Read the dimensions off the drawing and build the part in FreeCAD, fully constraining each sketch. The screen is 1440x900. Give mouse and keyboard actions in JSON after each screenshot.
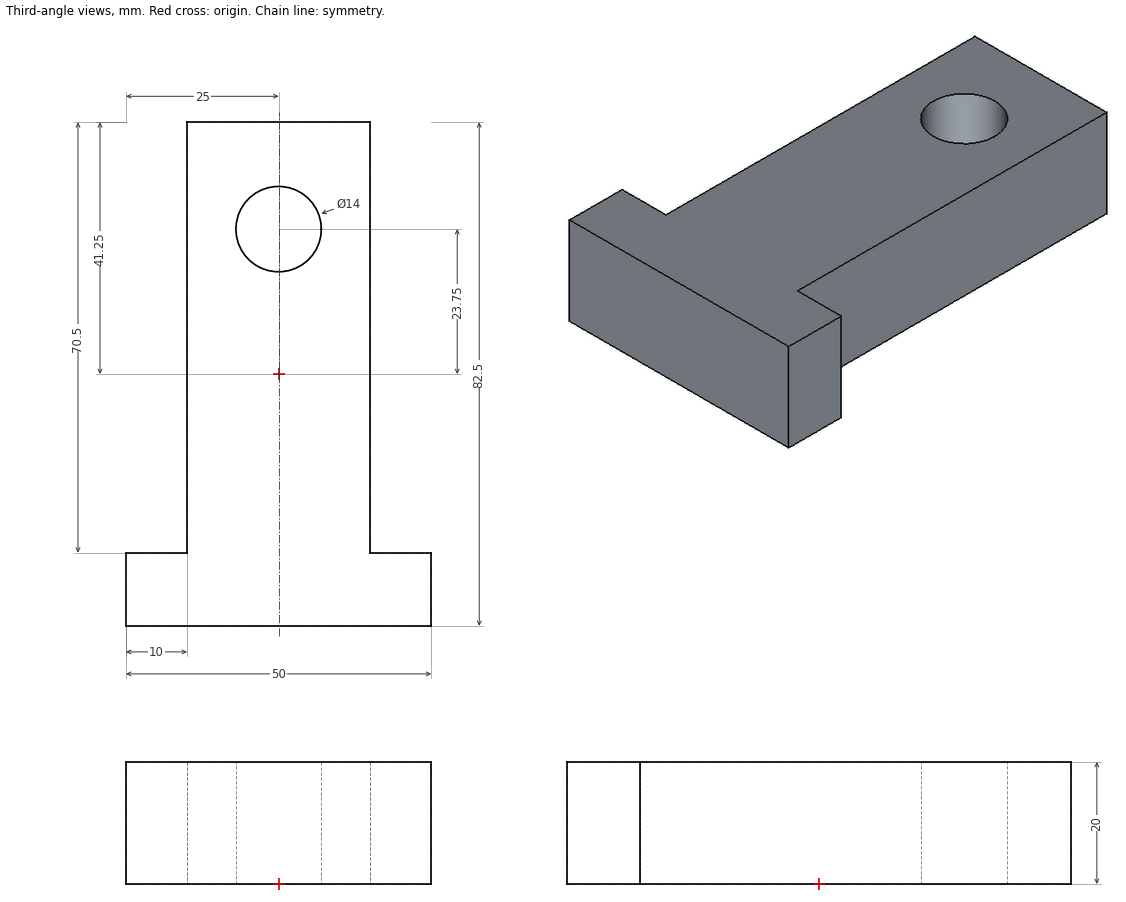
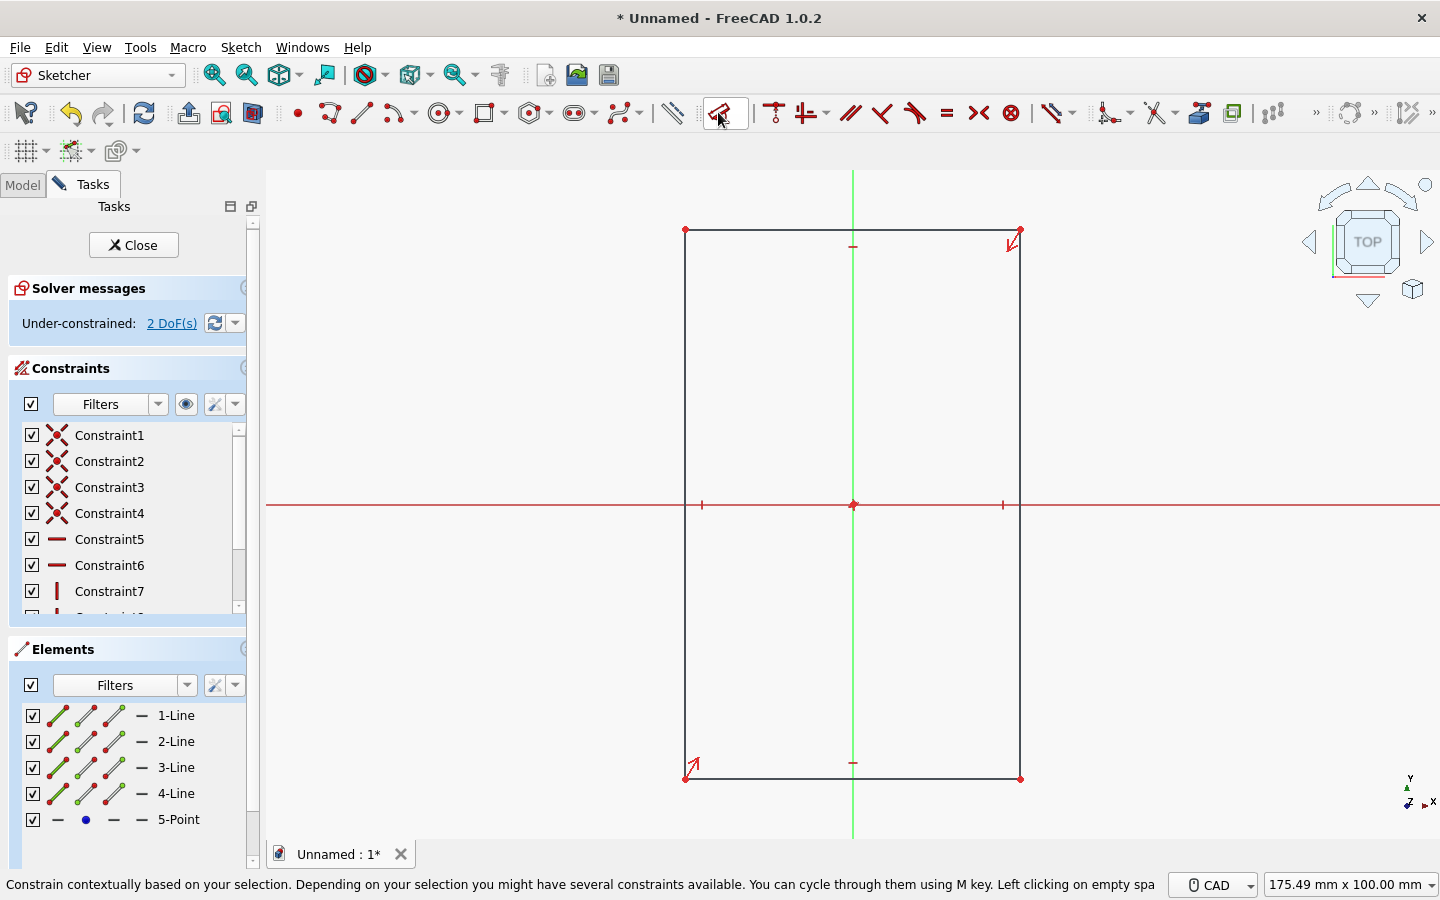
{"action": "left_click", "coordinate": [786, 779]}
{"action": "left_click", "coordinate": [776, 745]}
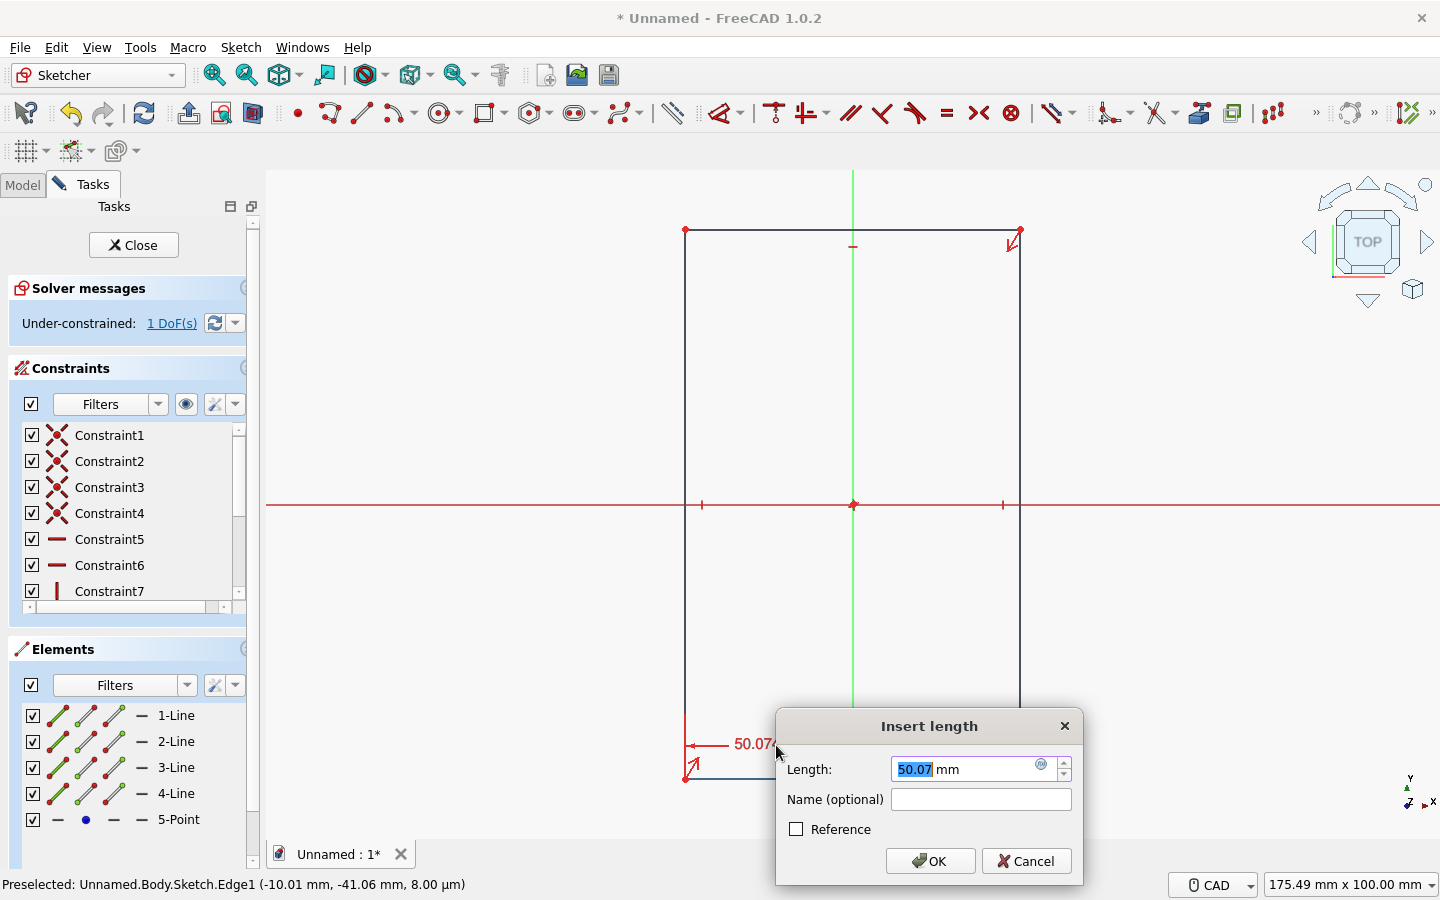
{"action": "type", "text": "50"}
{"action": "key", "text": "Return"}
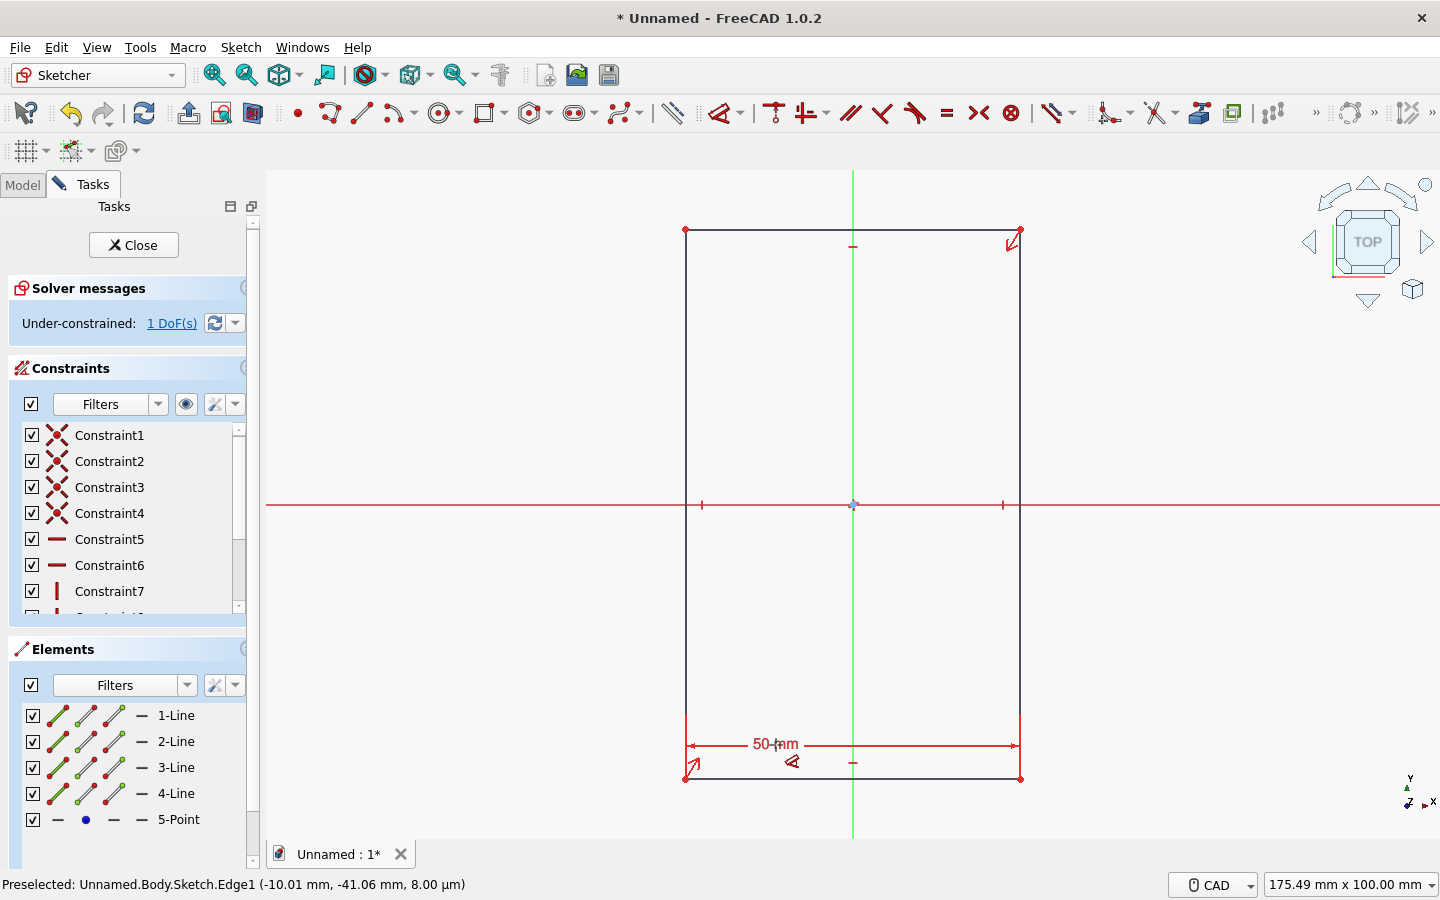
{"action": "left_click", "coordinate": [1020, 614]}
{"action": "left_click", "coordinate": [1054, 378]}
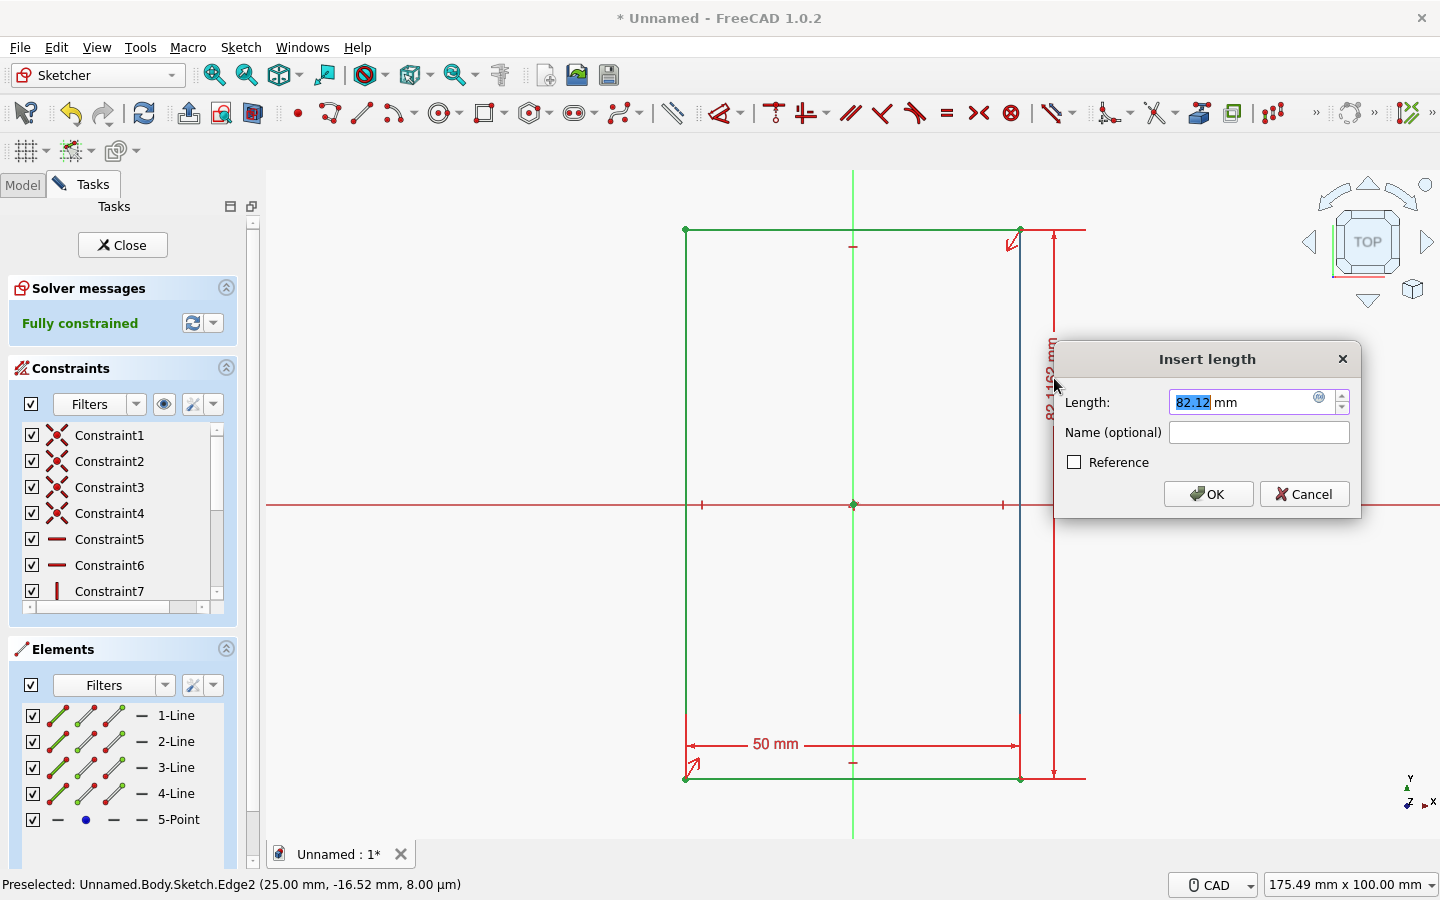
{"action": "type", "text": "82.5"}
{"action": "key", "text": "Return"}
{"action": "key", "text": "Escape"}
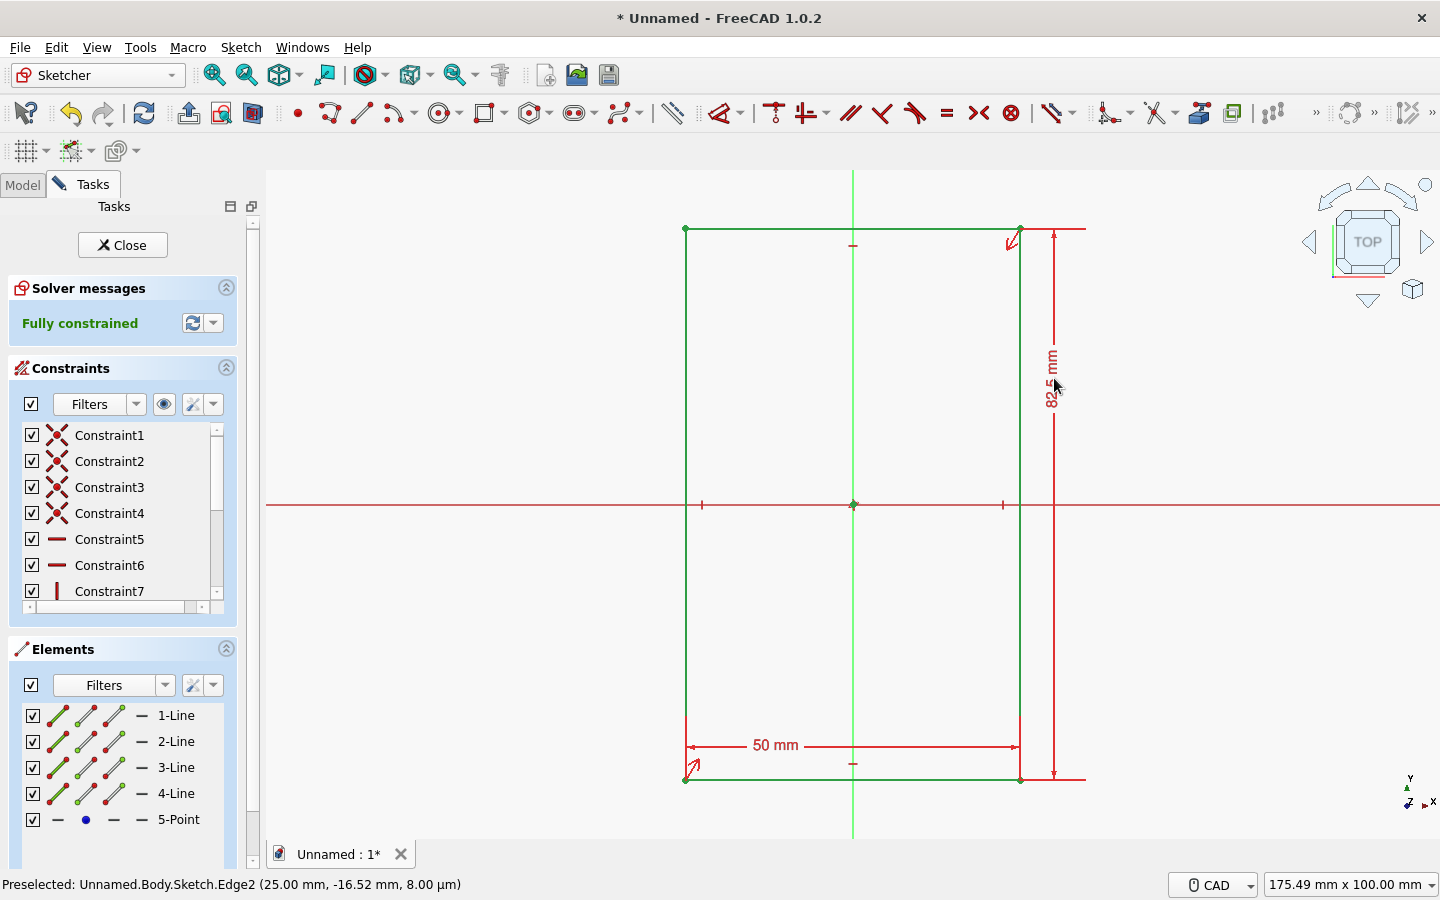
{"action": "left_click", "coordinate": [123, 245]}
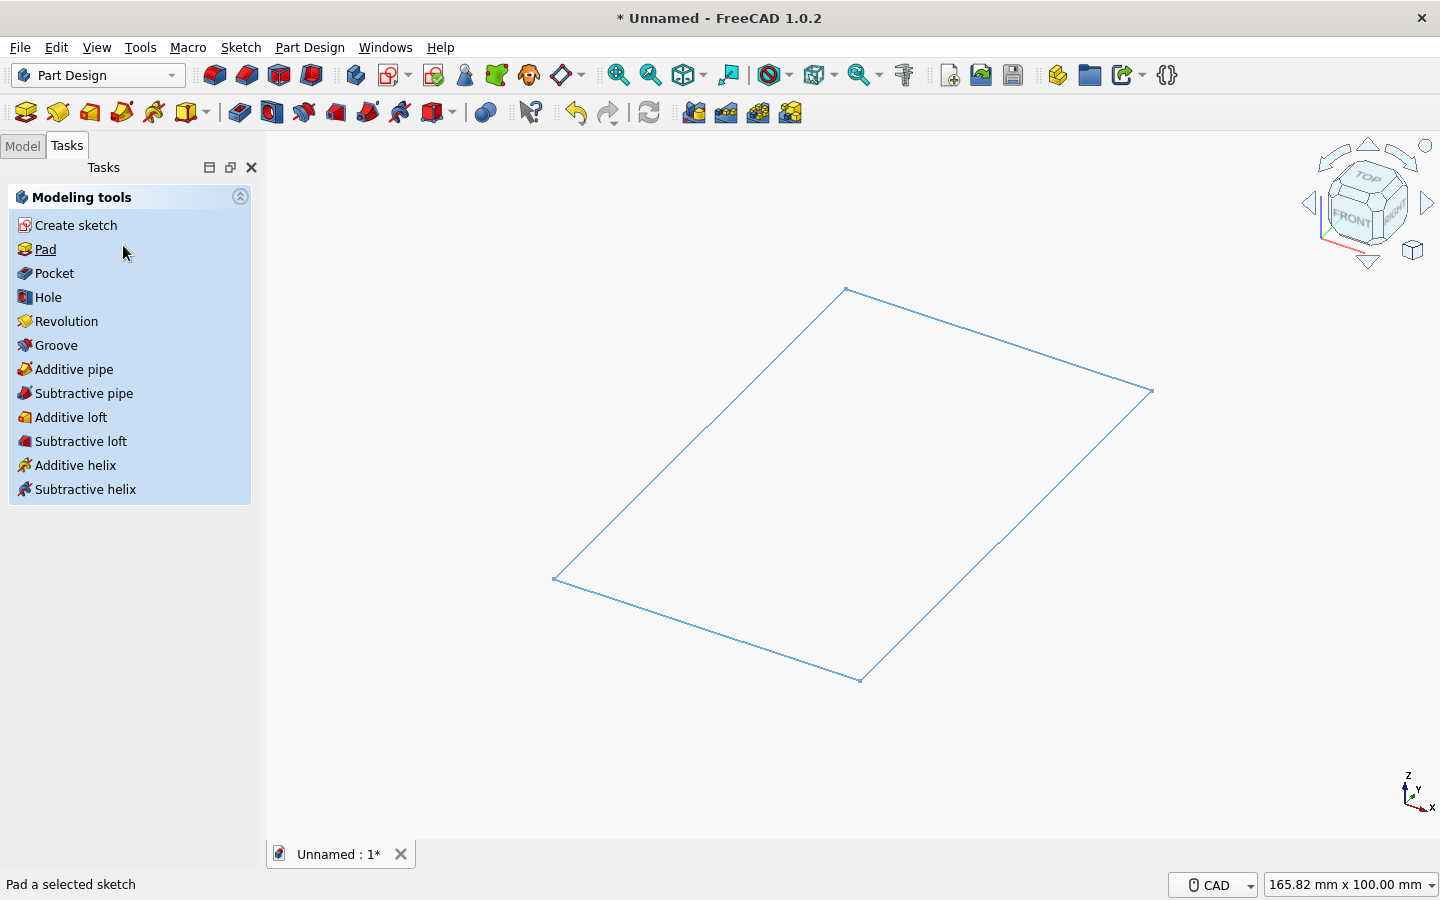
{"action": "left_click", "coordinate": [26, 112]}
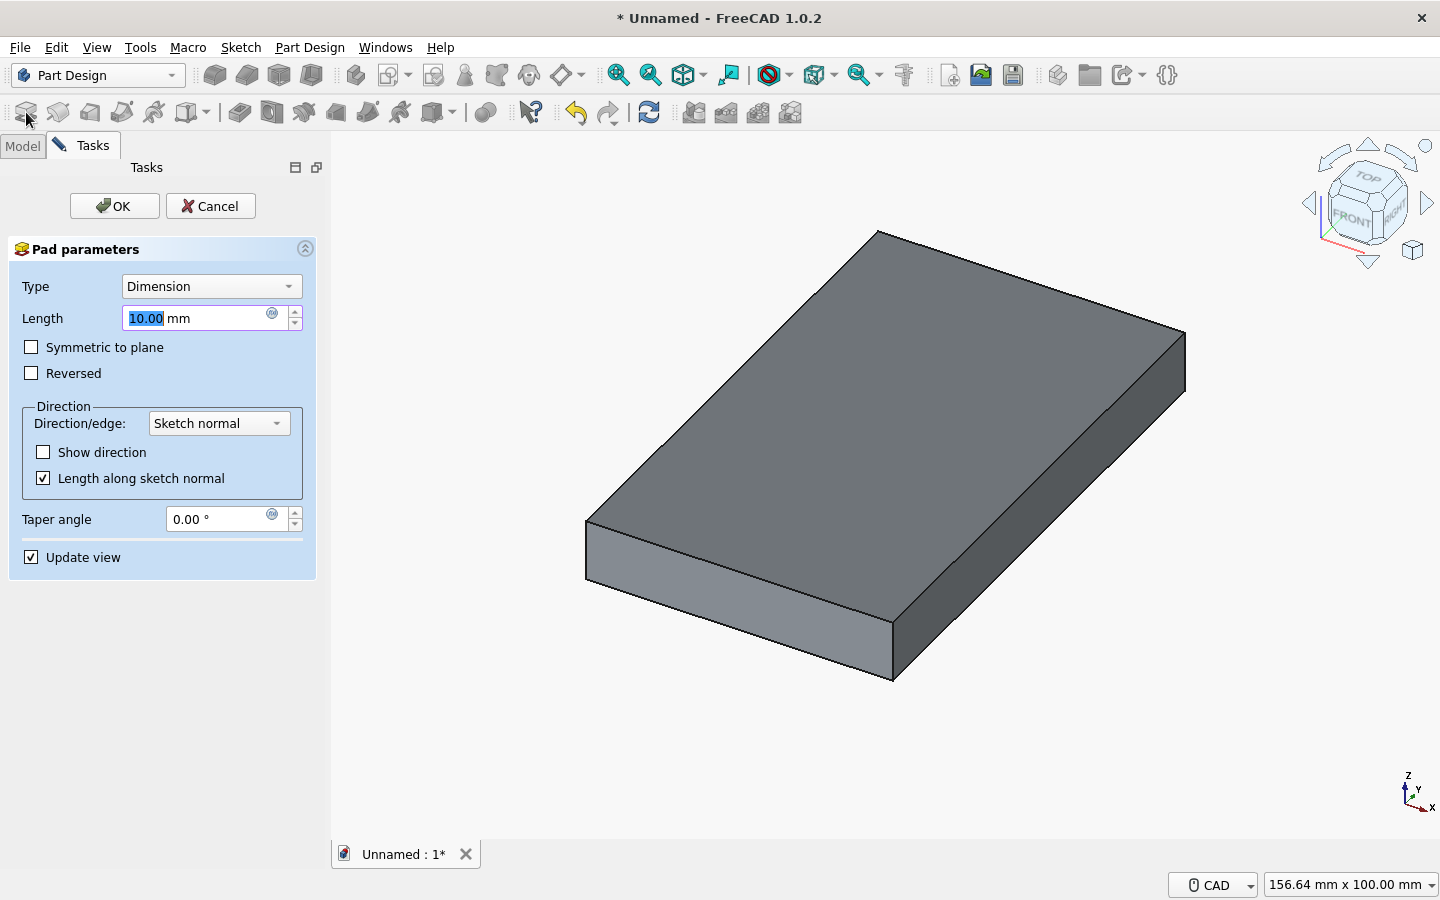
{"action": "type", "text": "20"}
{"action": "key", "text": "Tab"}